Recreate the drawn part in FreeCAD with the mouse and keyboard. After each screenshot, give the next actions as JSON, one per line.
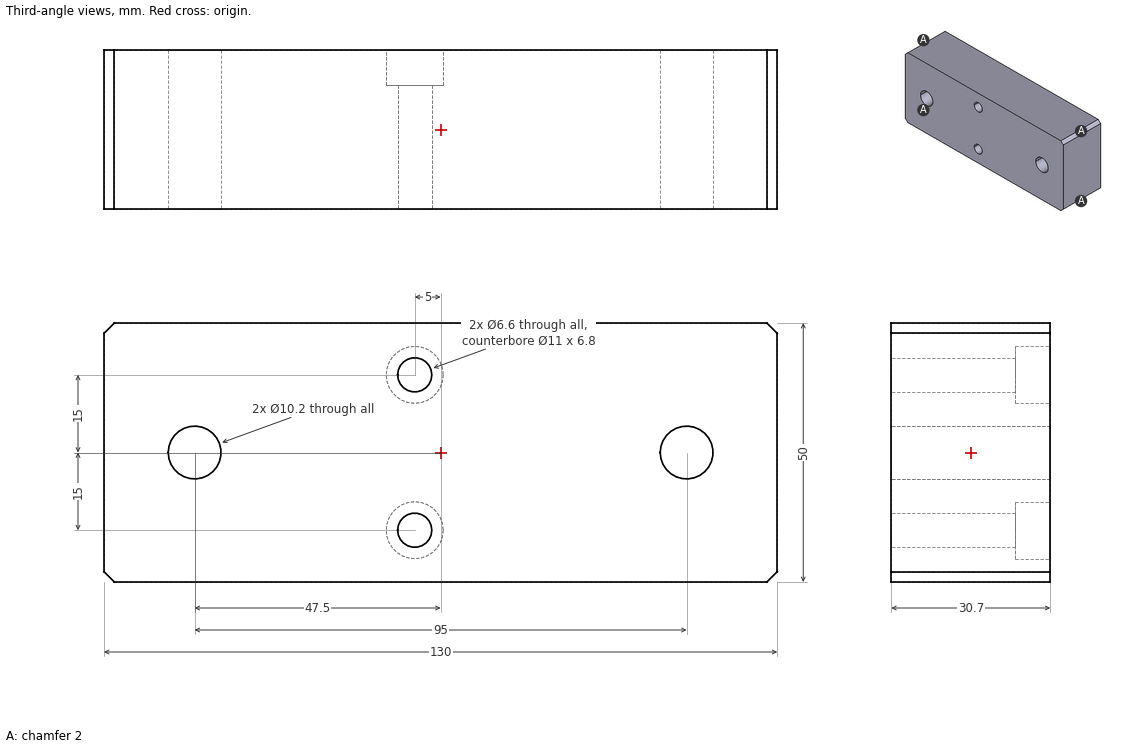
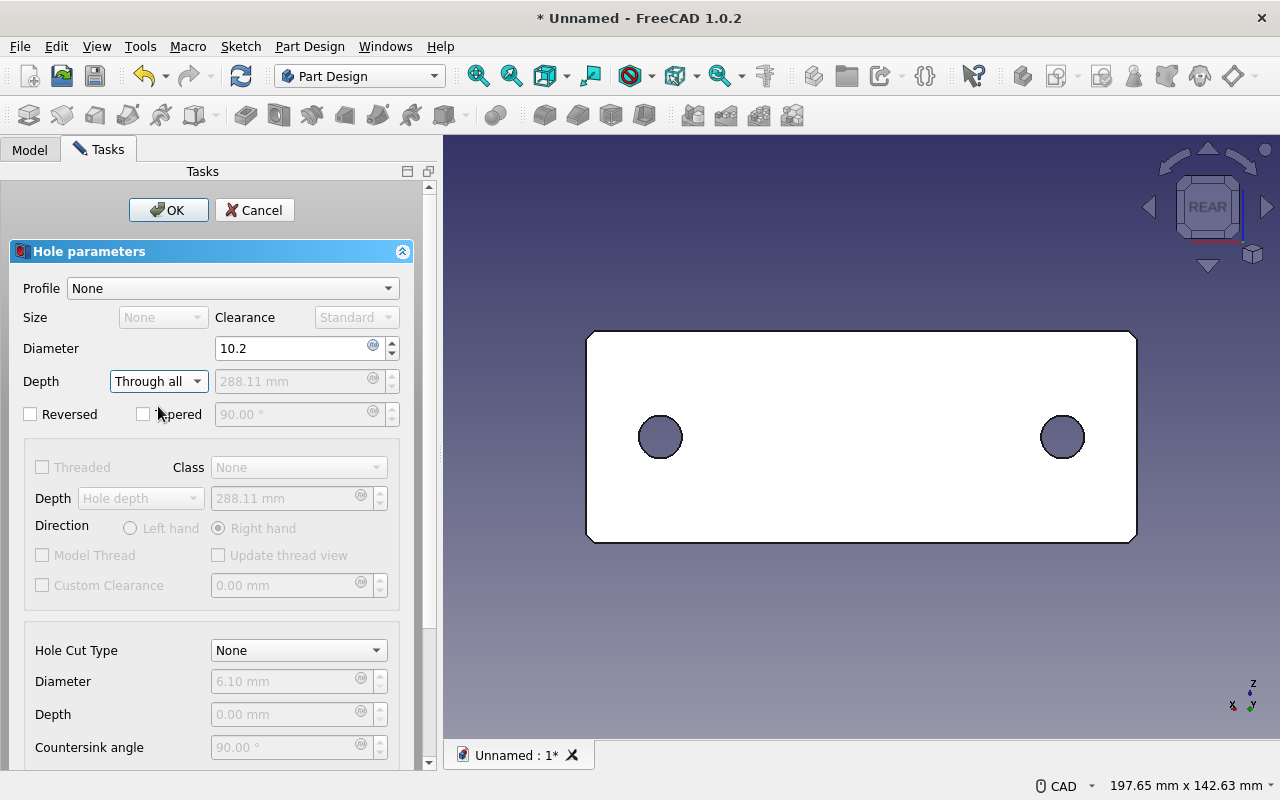
{"action": "left_click", "coordinate": [169, 210]}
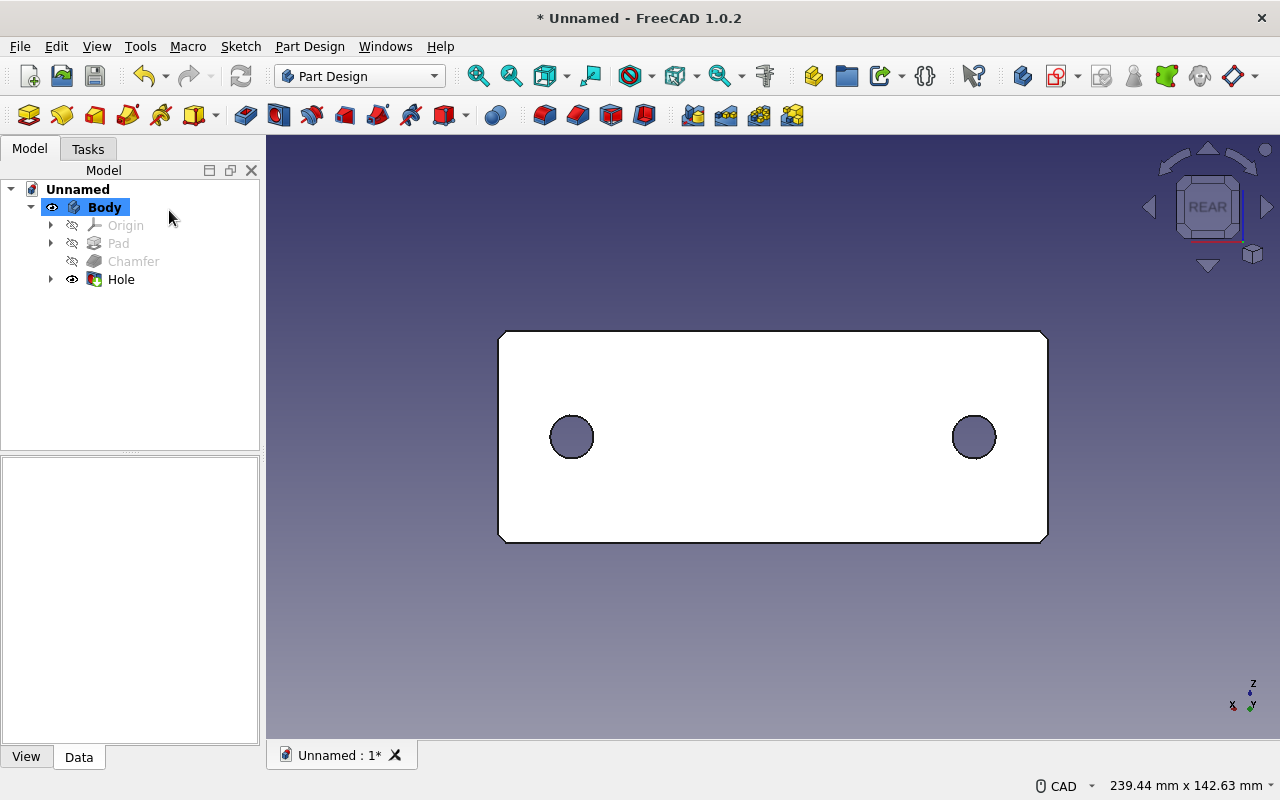
{"action": "left_click", "coordinate": [773, 436]}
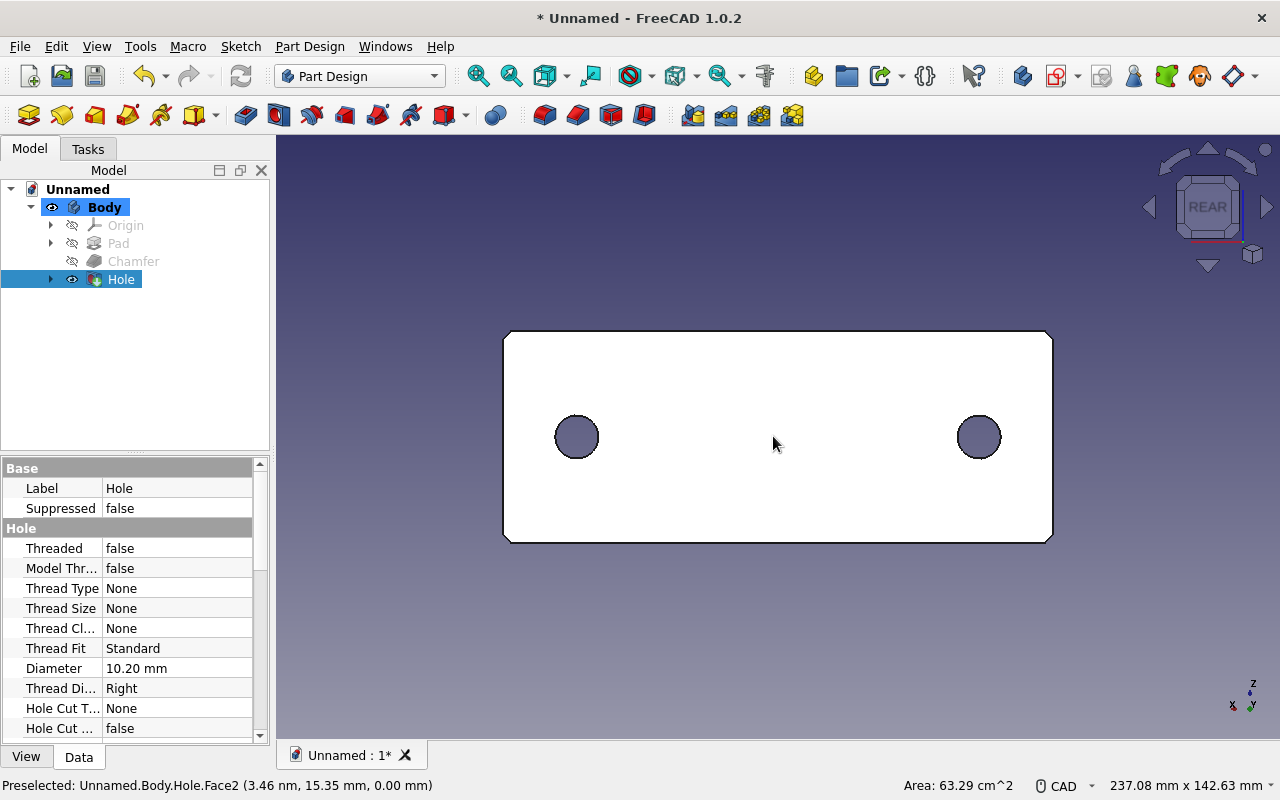
{"action": "left_click", "coordinate": [1056, 76]}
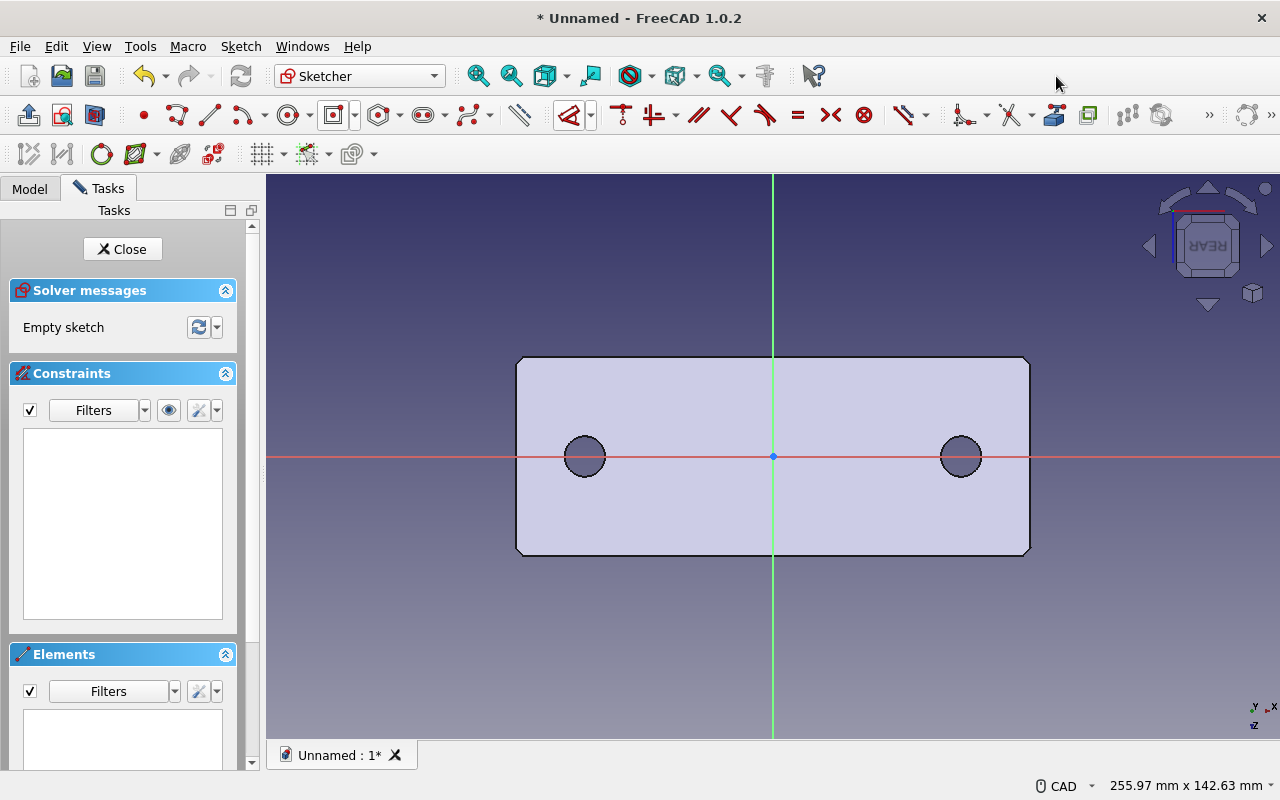
{"action": "scroll", "coordinate": [787, 456], "scroll_direction": "up", "scroll_amount": 5}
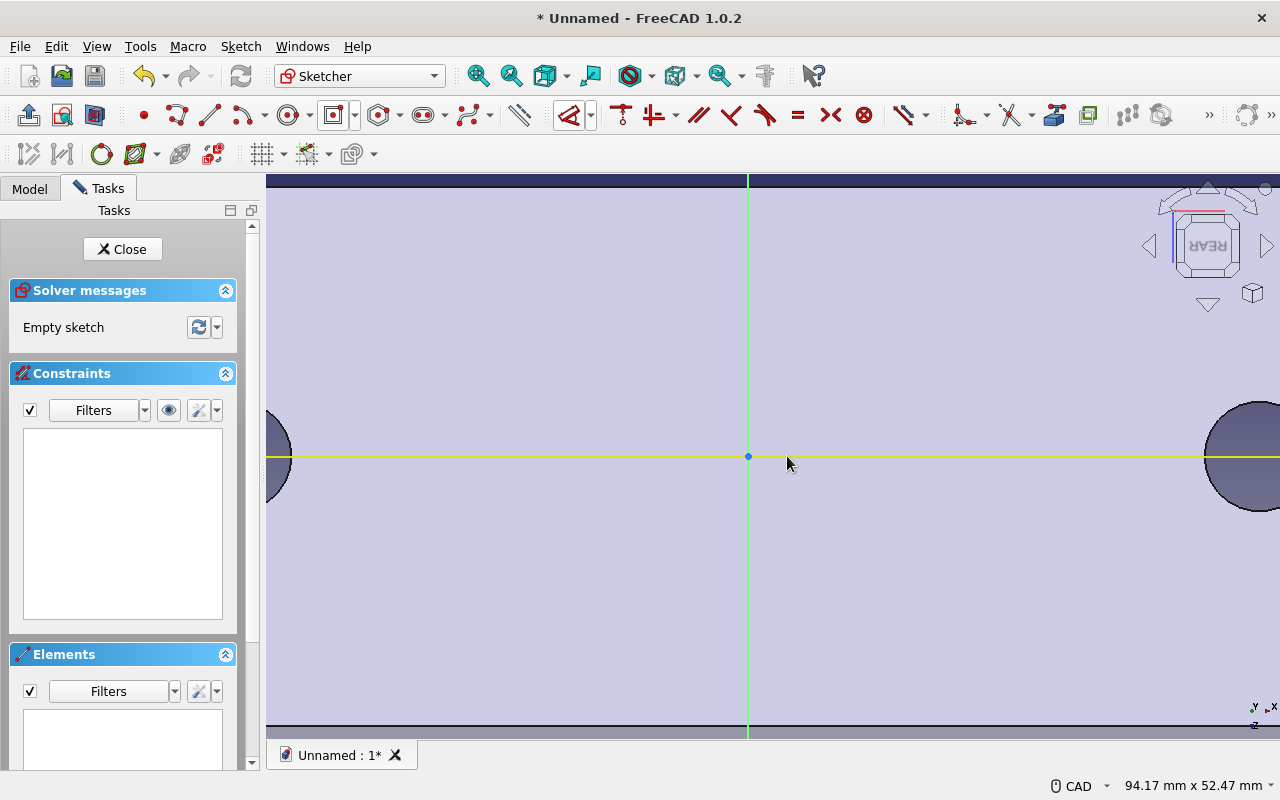
{"action": "left_click", "coordinate": [288, 116]}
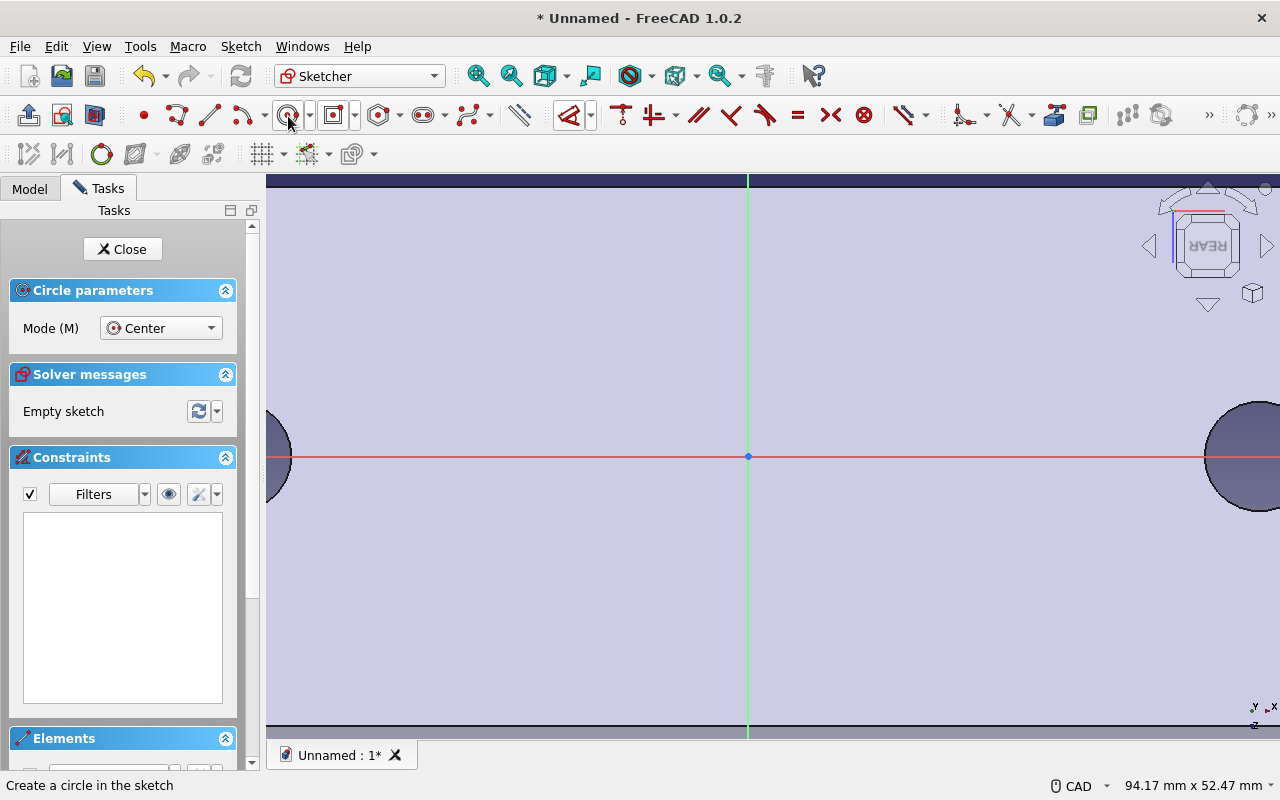
{"action": "left_click", "coordinate": [694, 618]}
{"action": "left_click", "coordinate": [719, 593]}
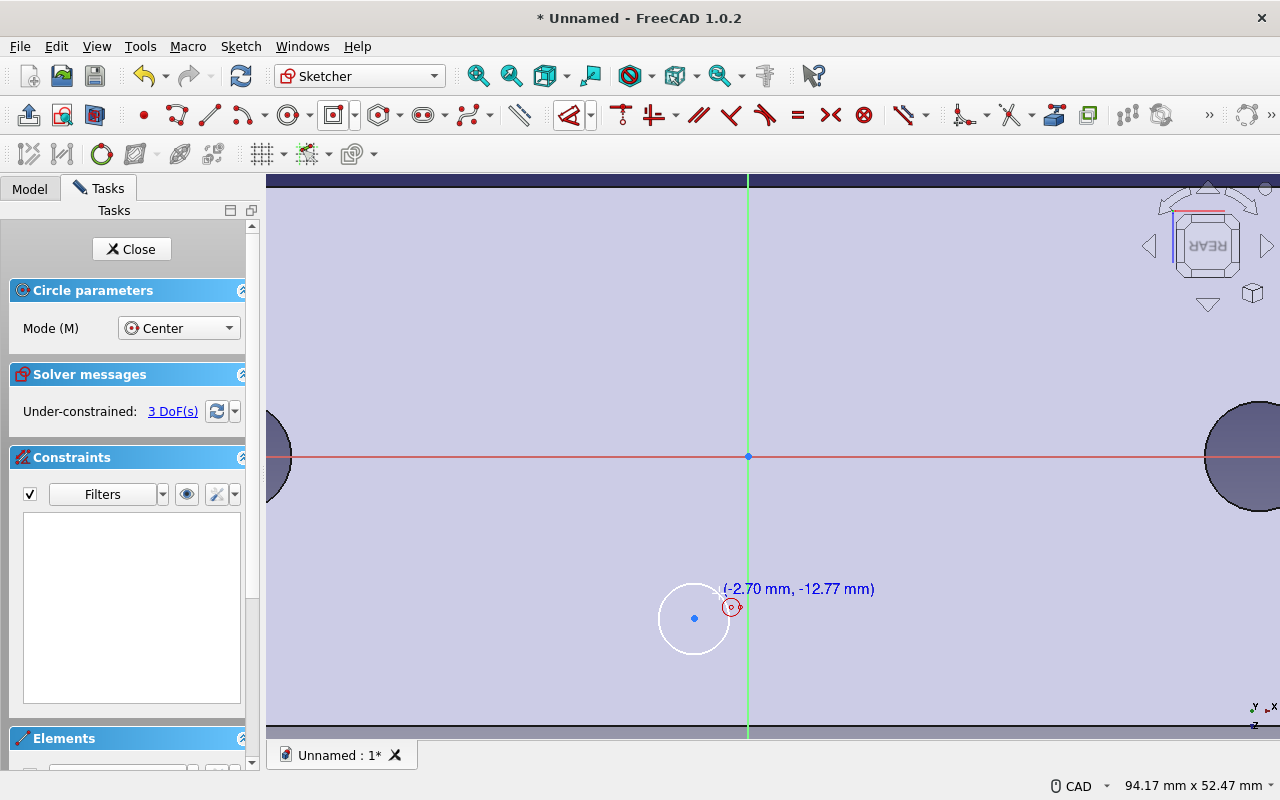
{"action": "left_click", "coordinate": [694, 295]}
{"action": "left_click", "coordinate": [719, 270]}
{"action": "key", "text": "Escape"}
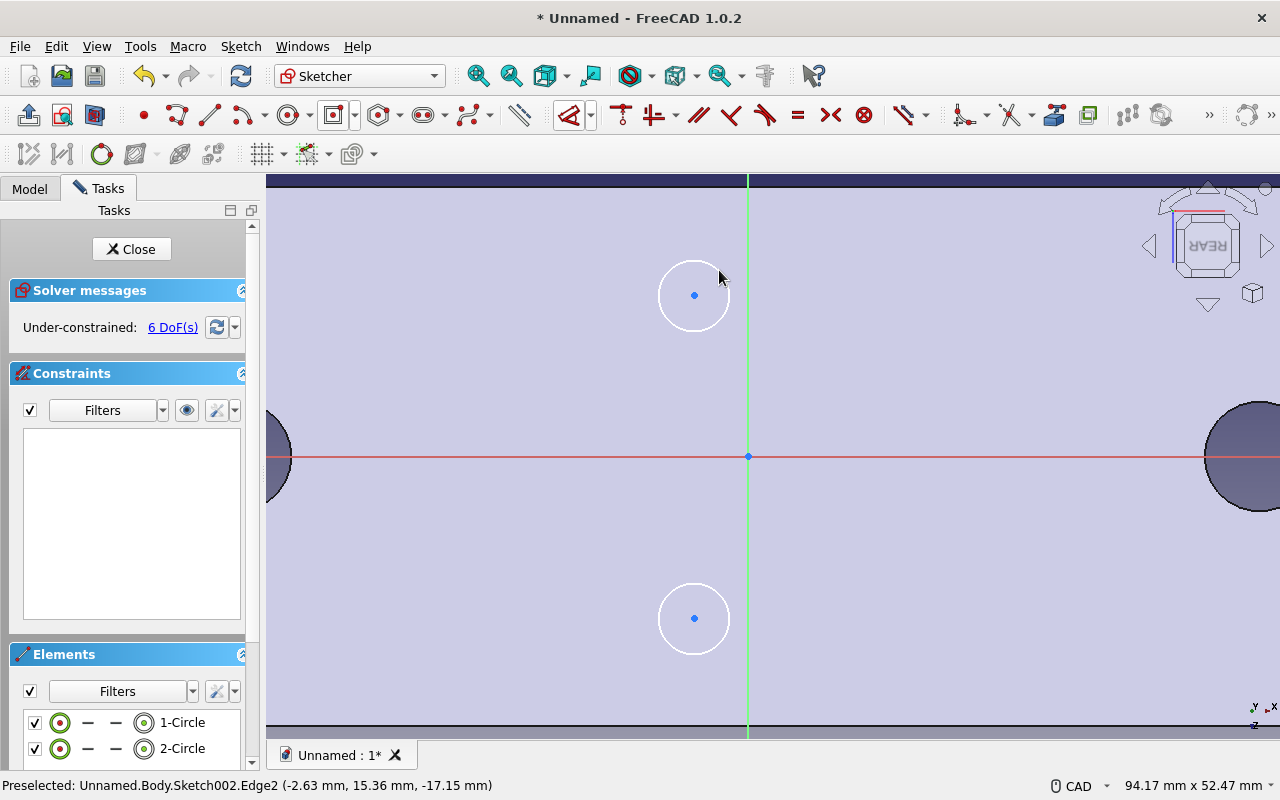
{"action": "left_click", "coordinate": [719, 594]}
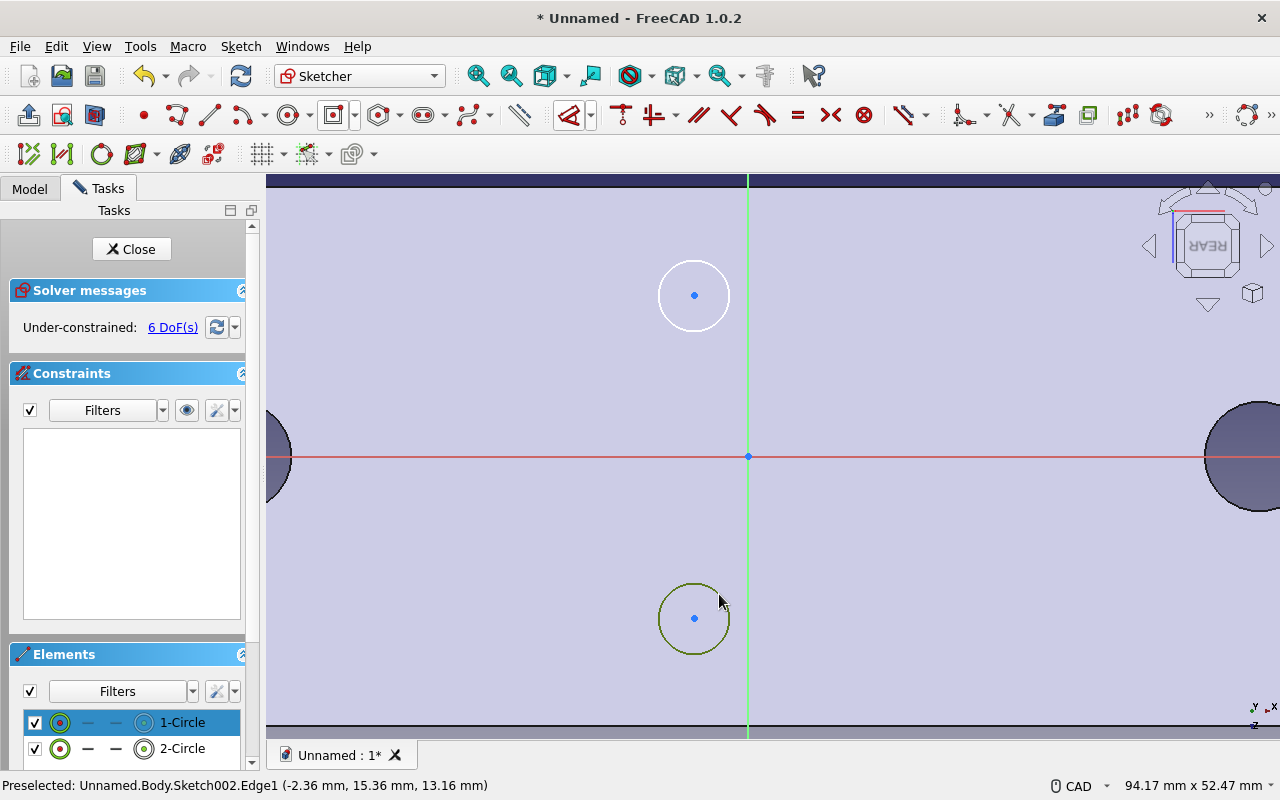
{"action": "left_click", "coordinate": [719, 271]}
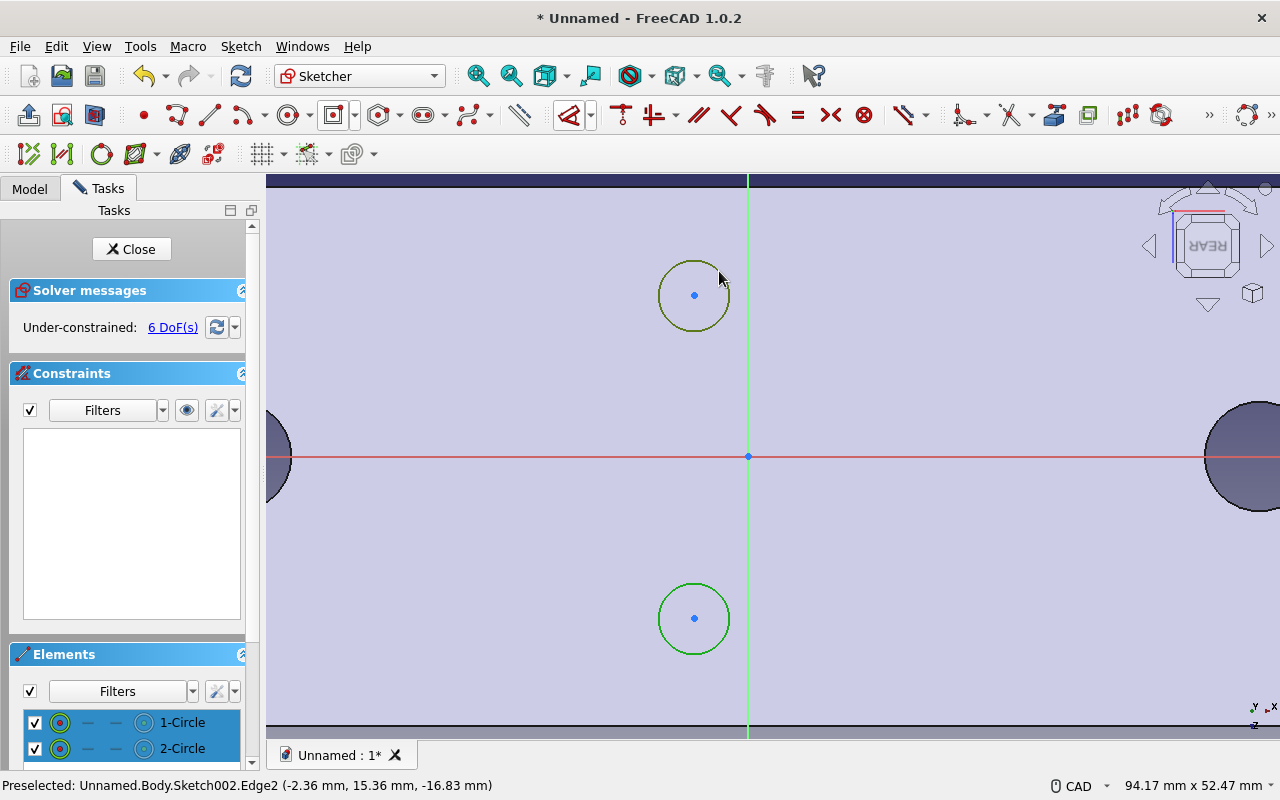
{"action": "left_click", "coordinate": [798, 116]}